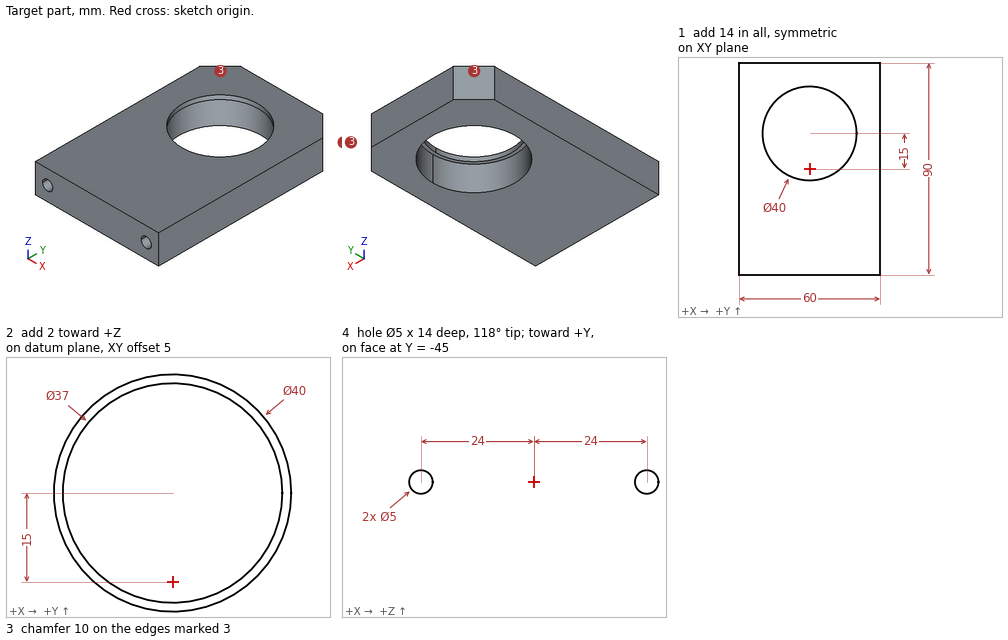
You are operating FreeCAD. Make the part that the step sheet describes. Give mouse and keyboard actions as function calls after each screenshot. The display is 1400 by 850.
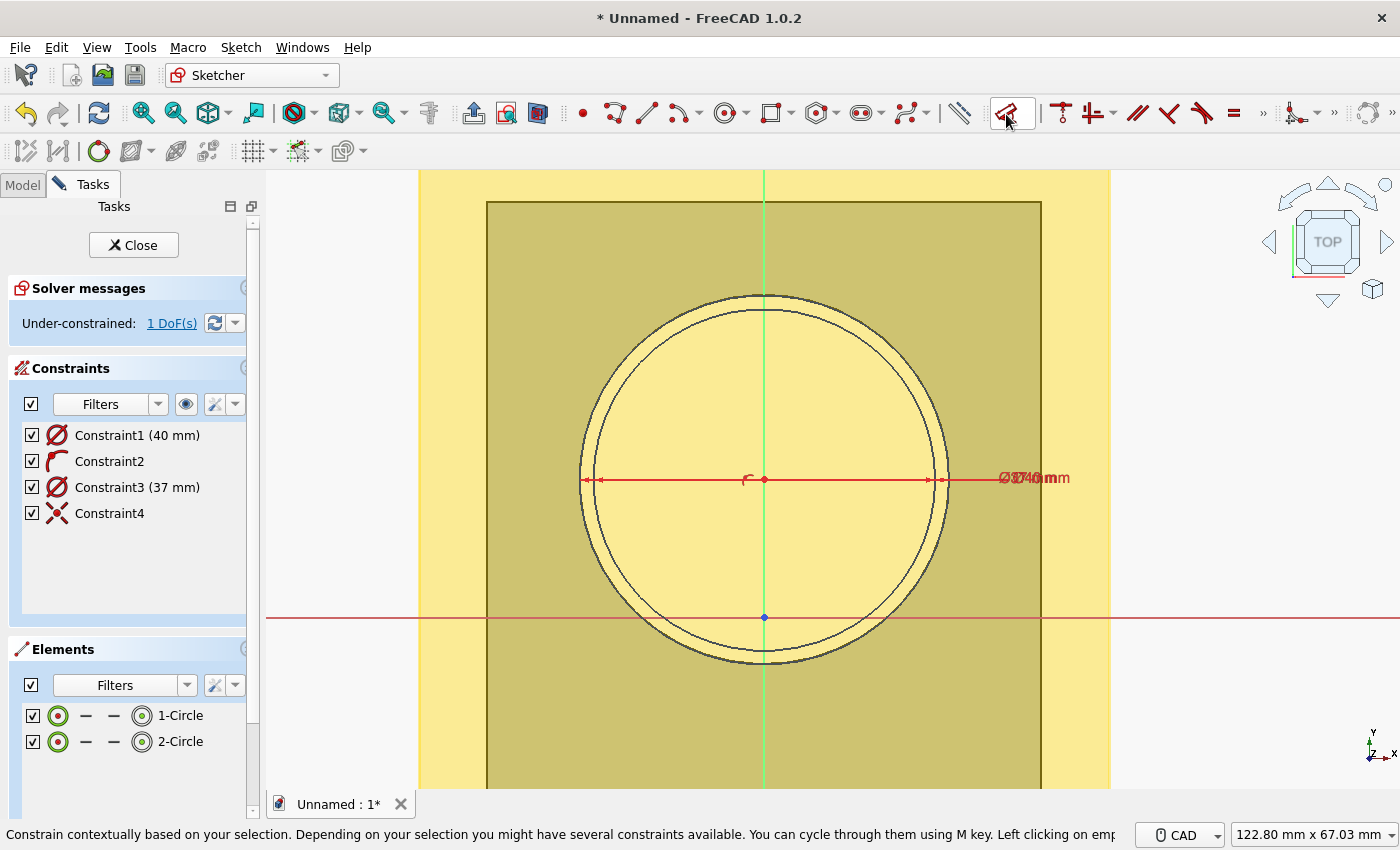
click(764, 480)
click(798, 549)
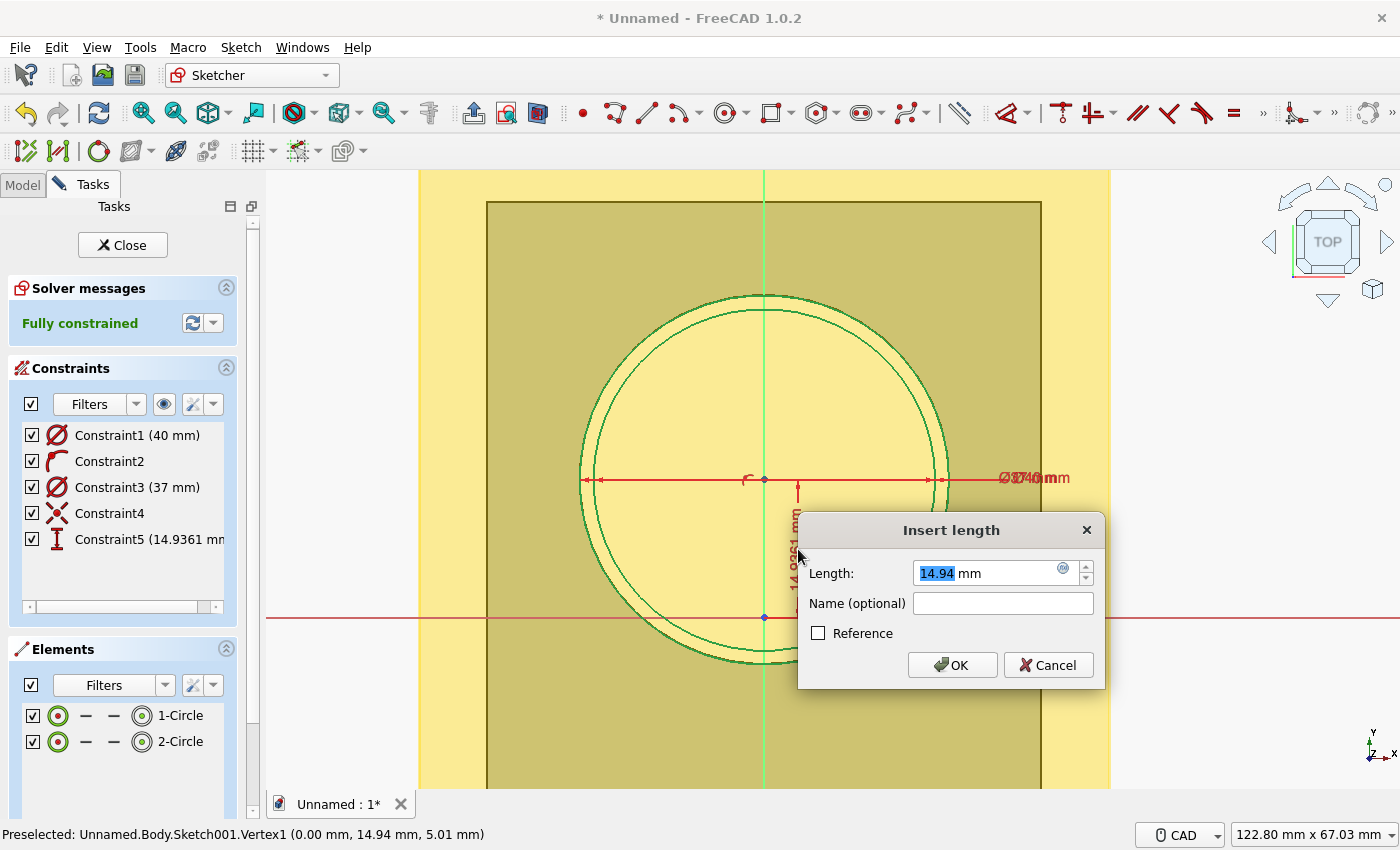
text(15)
key(Return)
key(Escape)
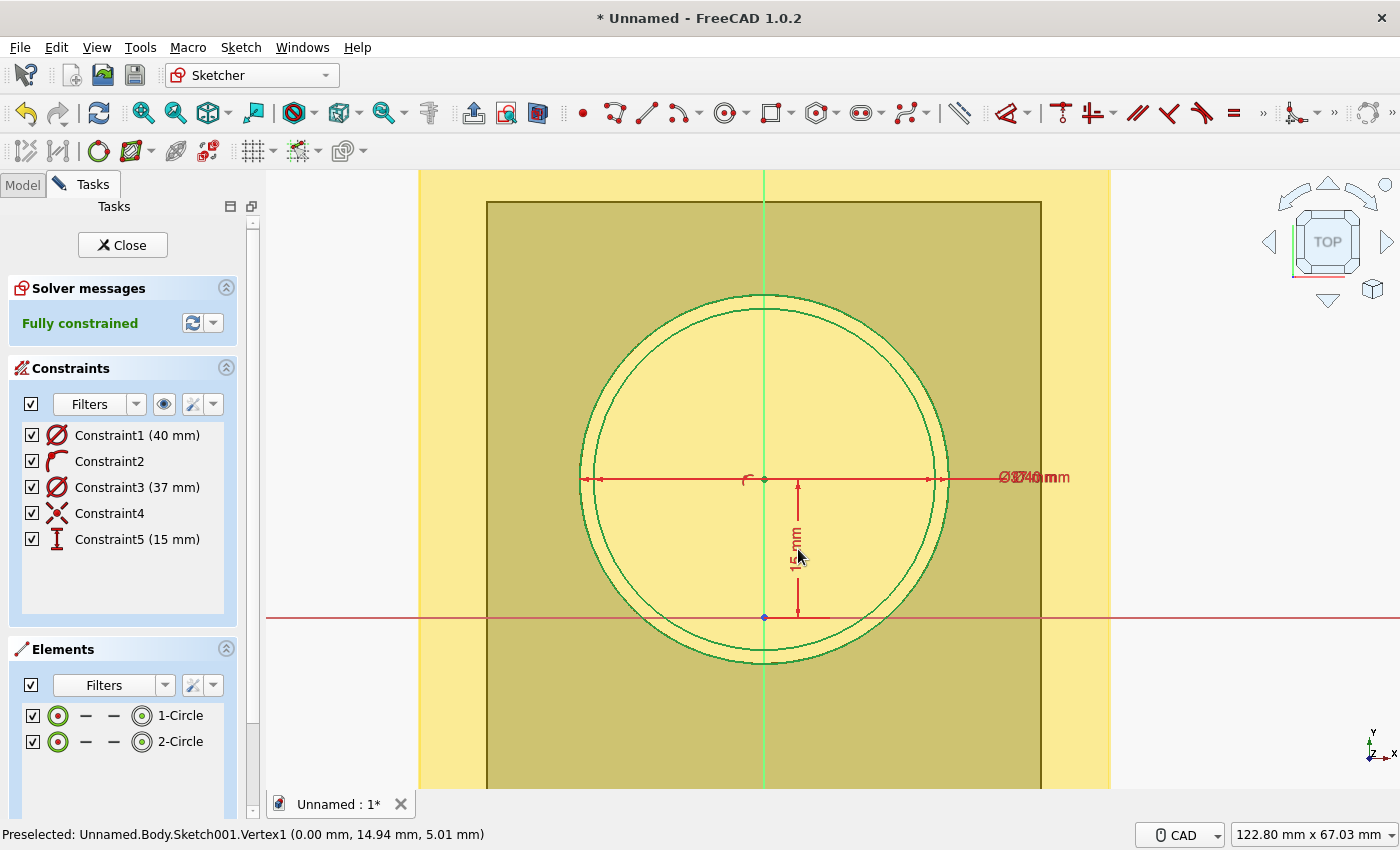
click(123, 245)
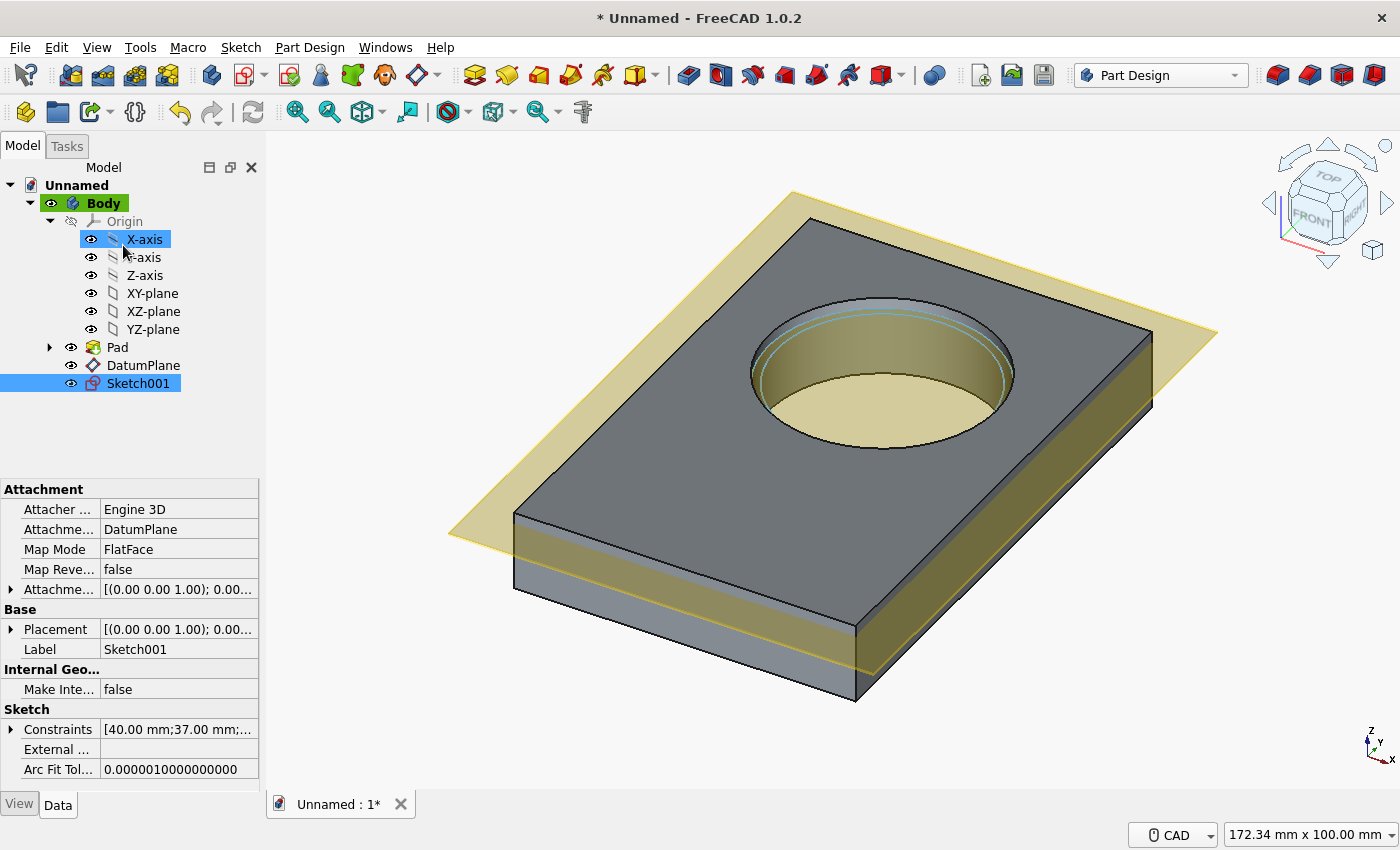
click(476, 76)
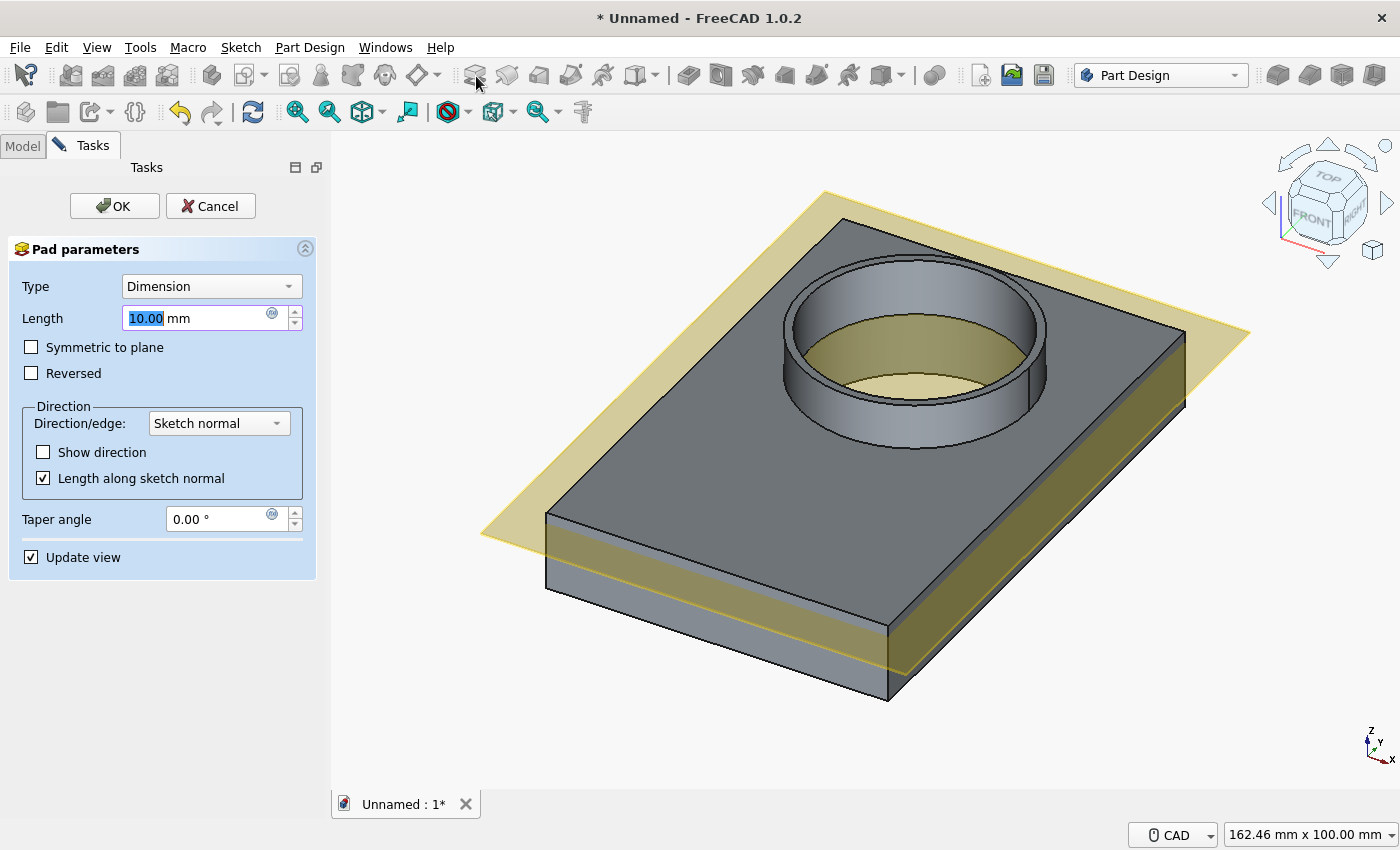
text(2)
key(Tab)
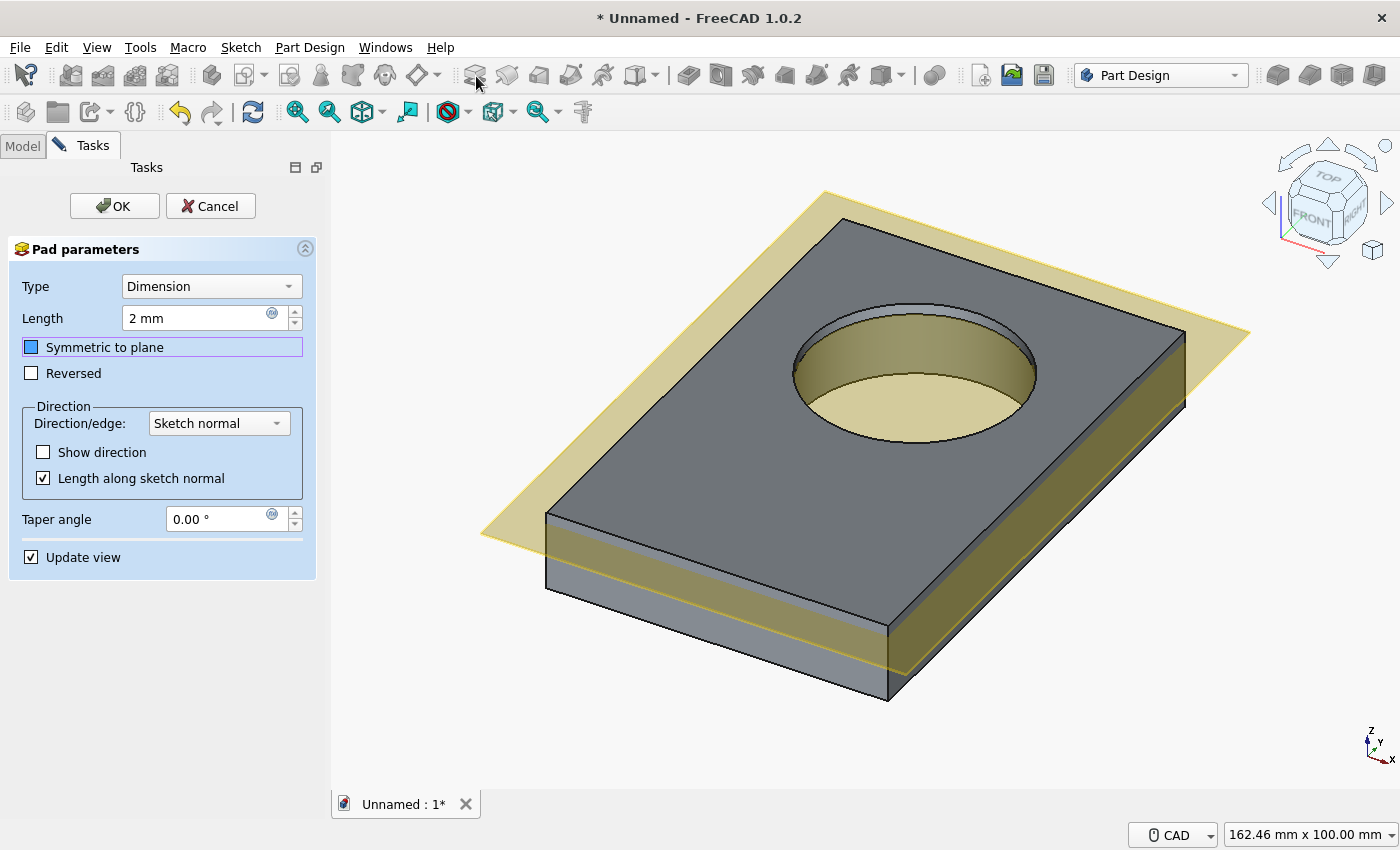
click(115, 206)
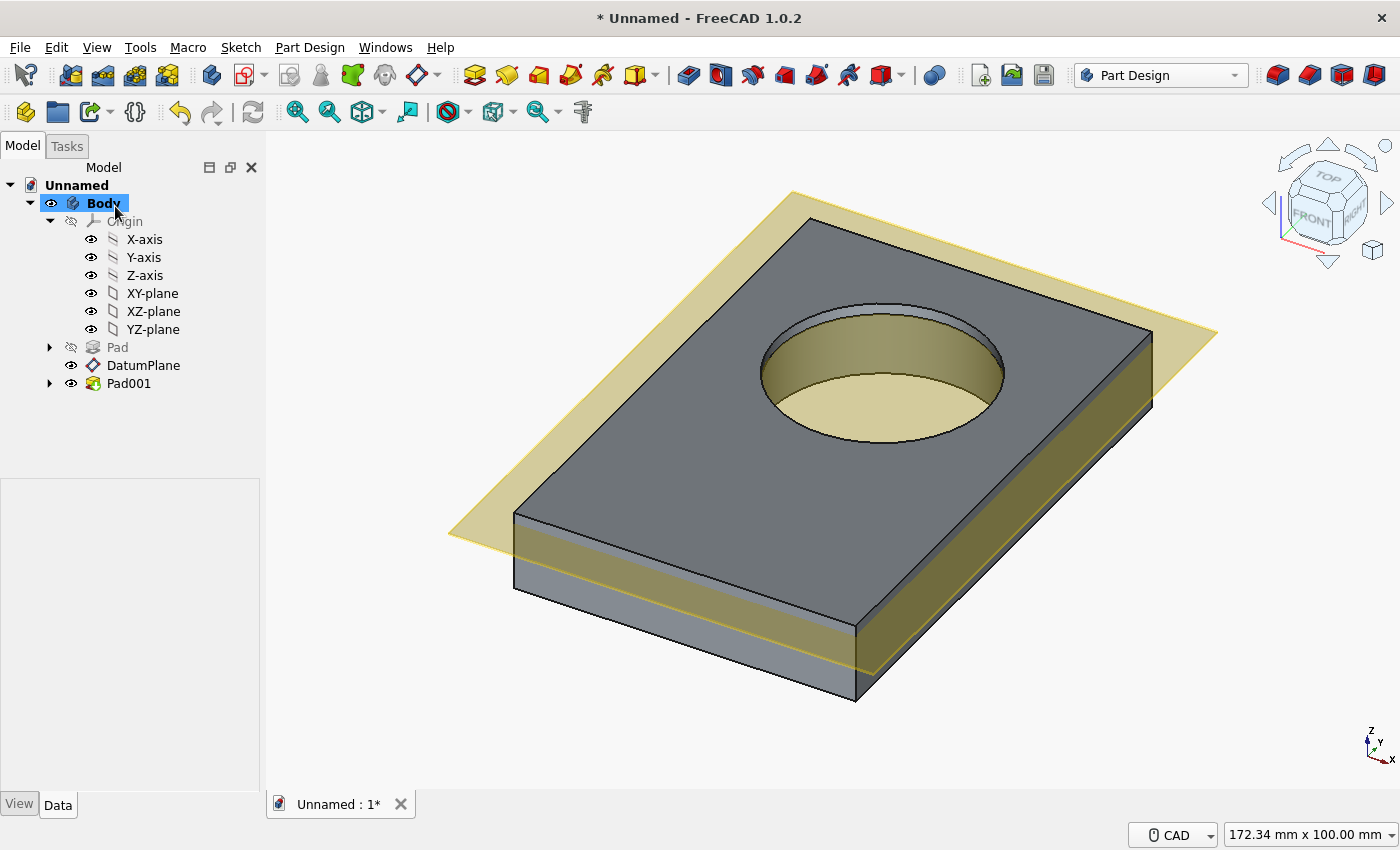
click(116, 365)
key(space)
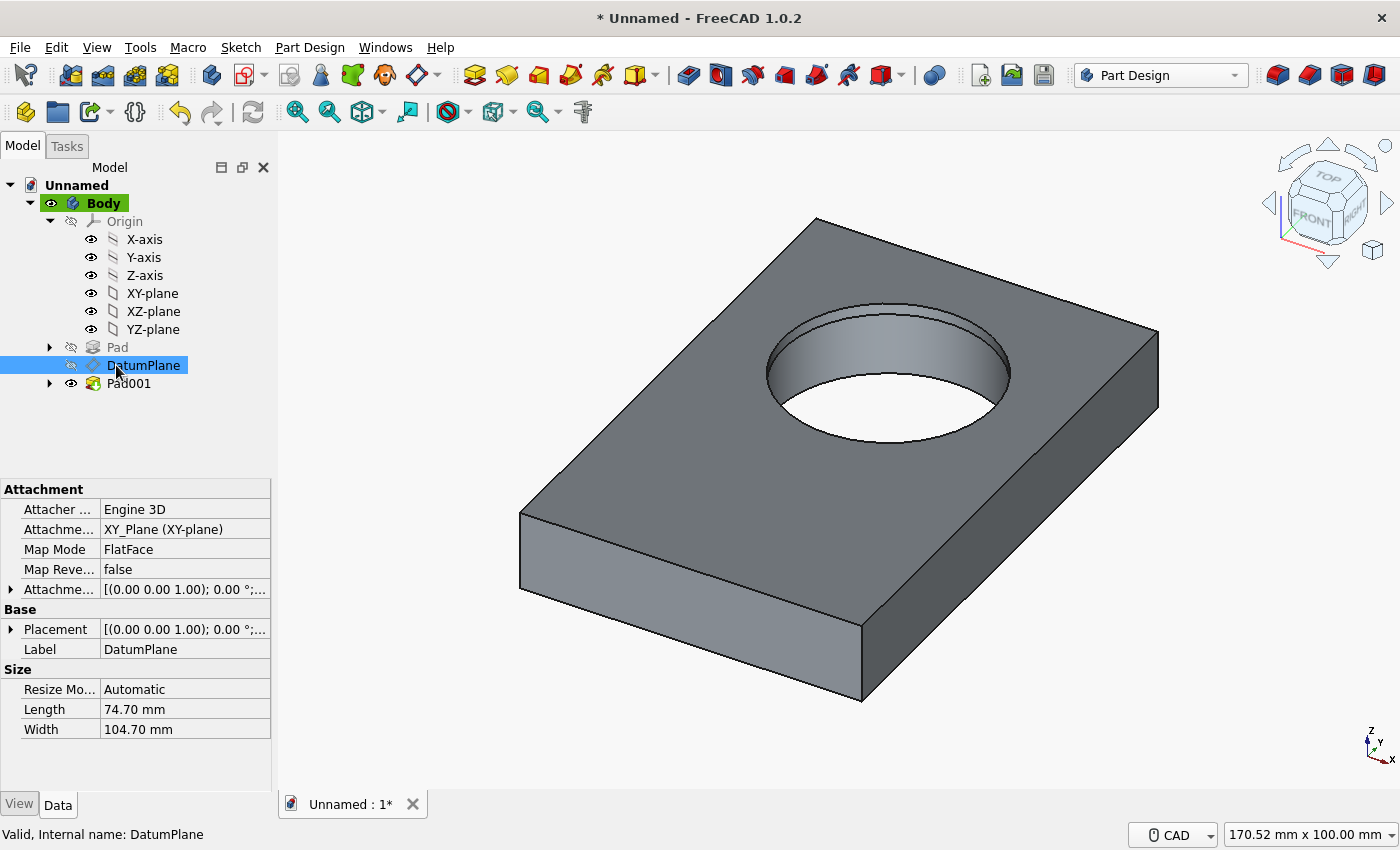
key(0)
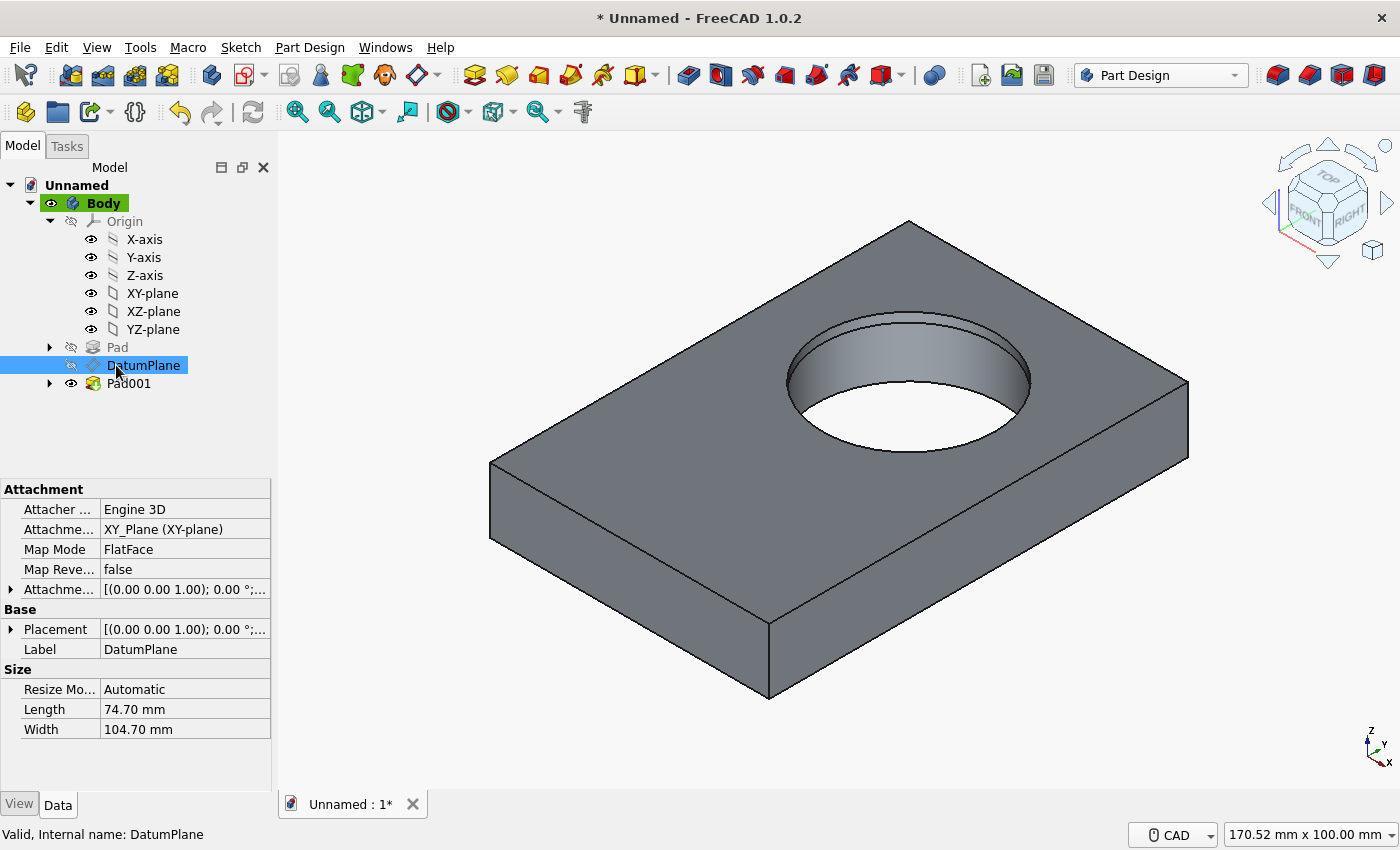
key(2)